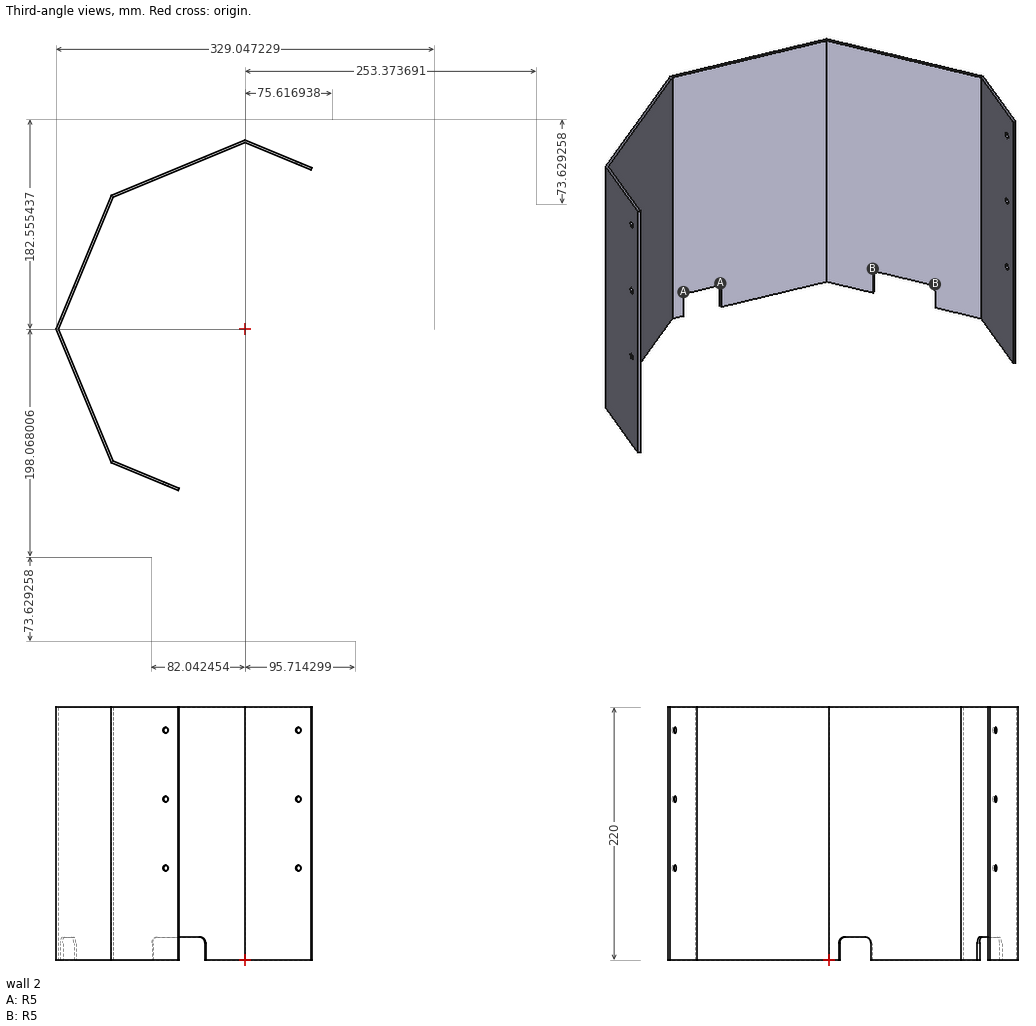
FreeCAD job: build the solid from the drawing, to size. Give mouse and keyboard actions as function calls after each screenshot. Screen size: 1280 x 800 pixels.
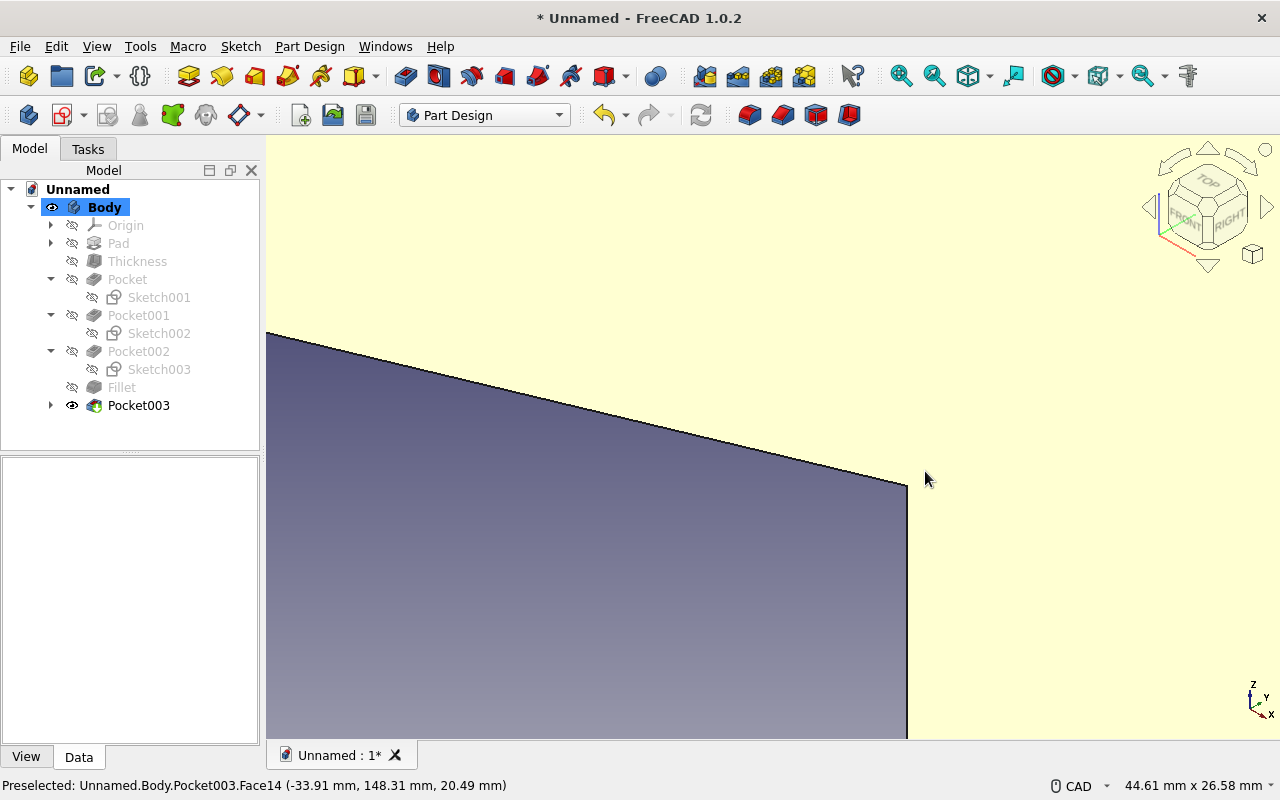
click(902, 76)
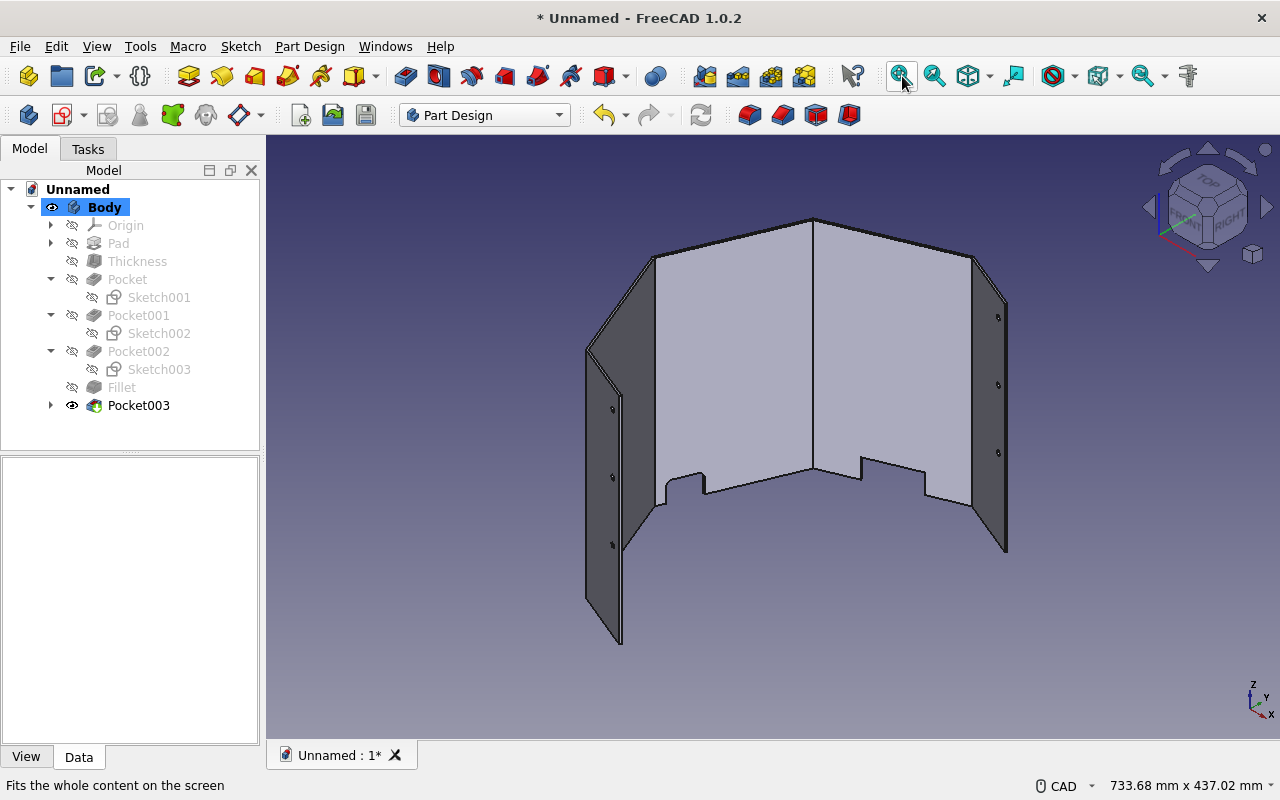
key(2)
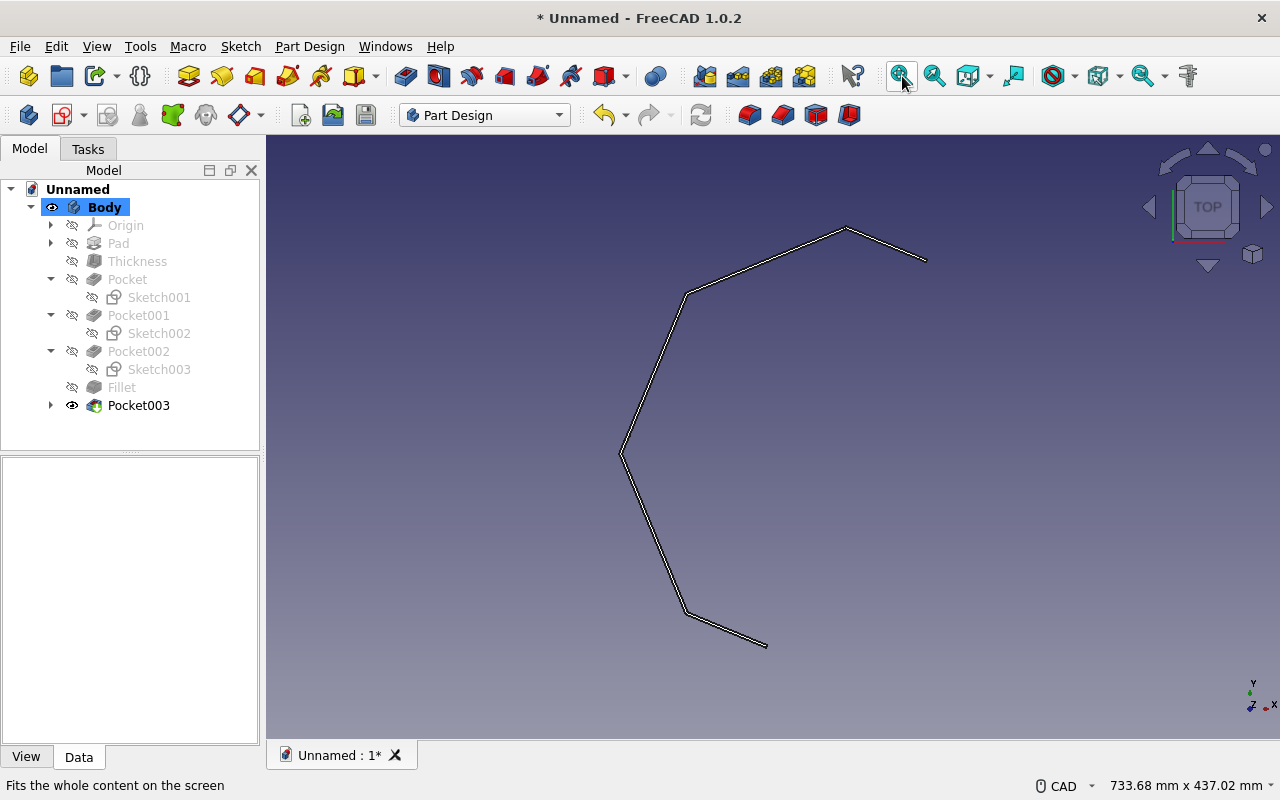
scroll(799, 247, up, 14)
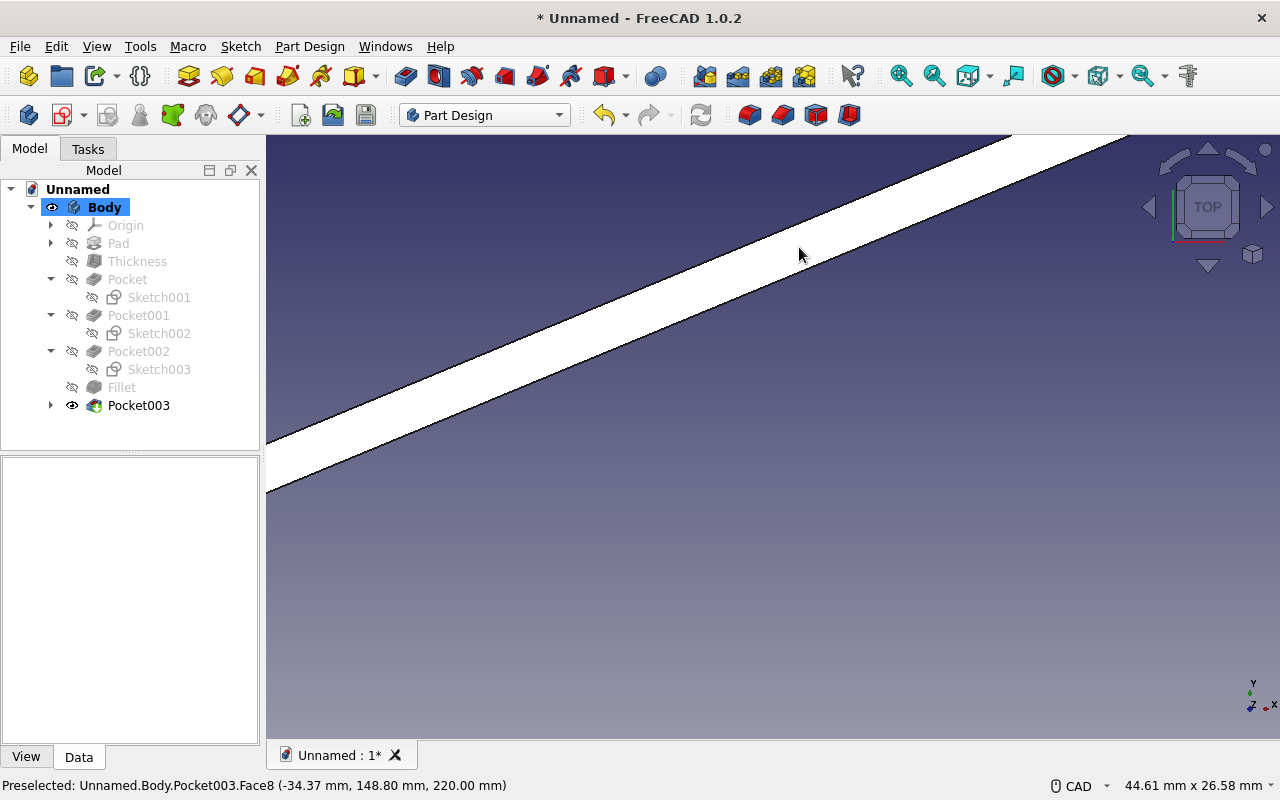
click(902, 76)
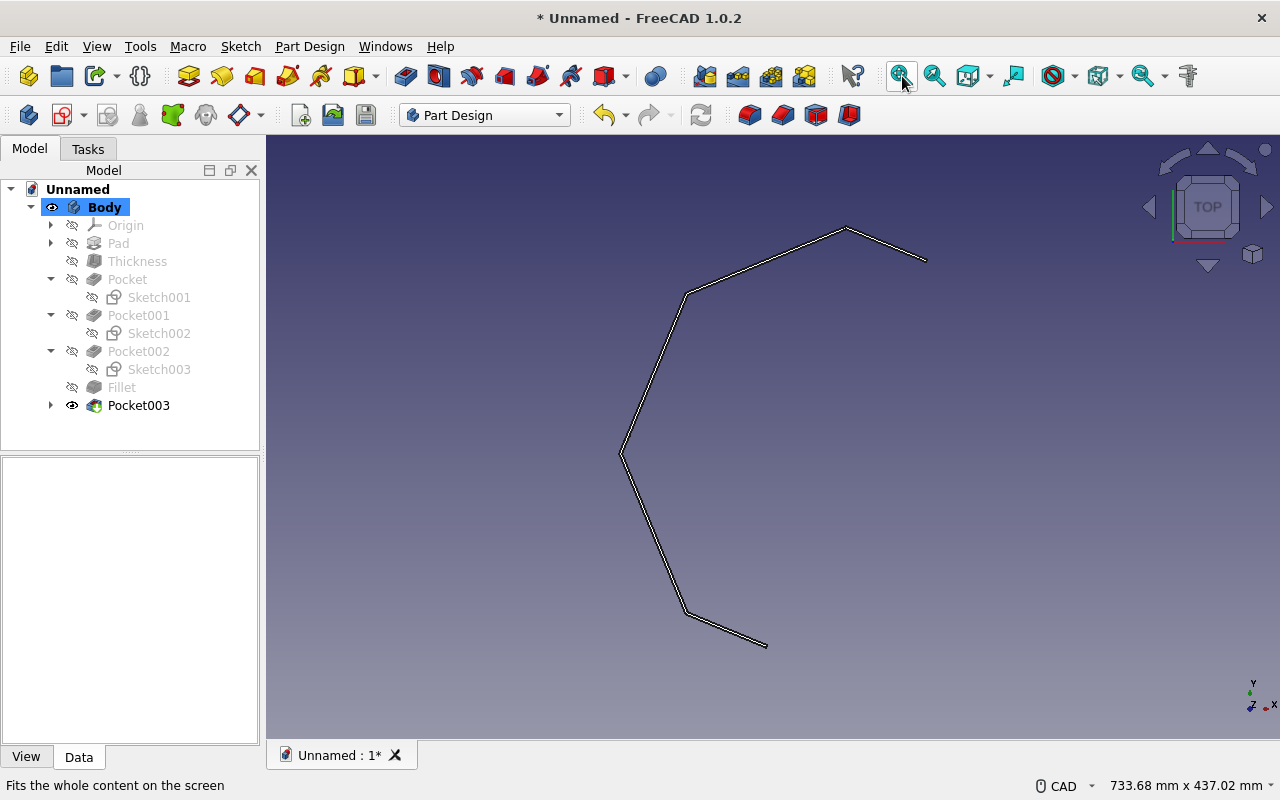
key(1)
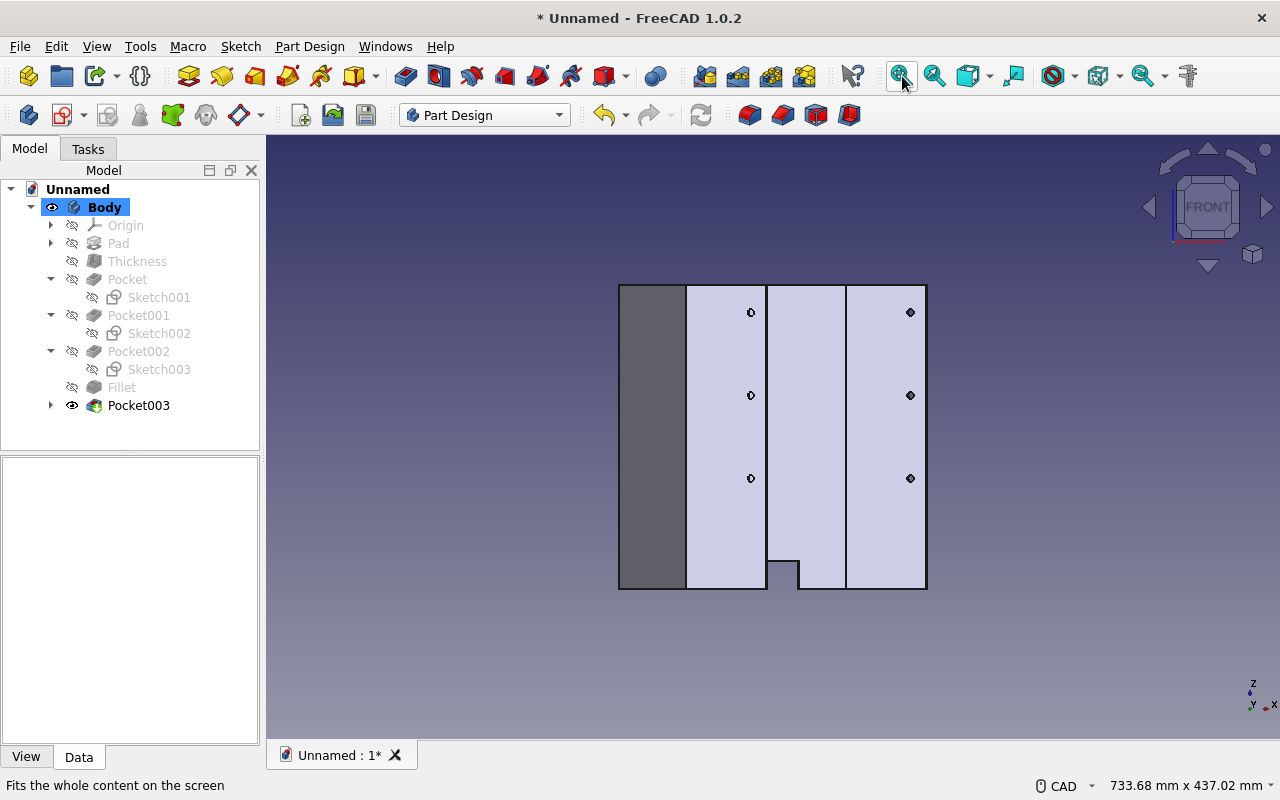
scroll(799, 560, up, 14)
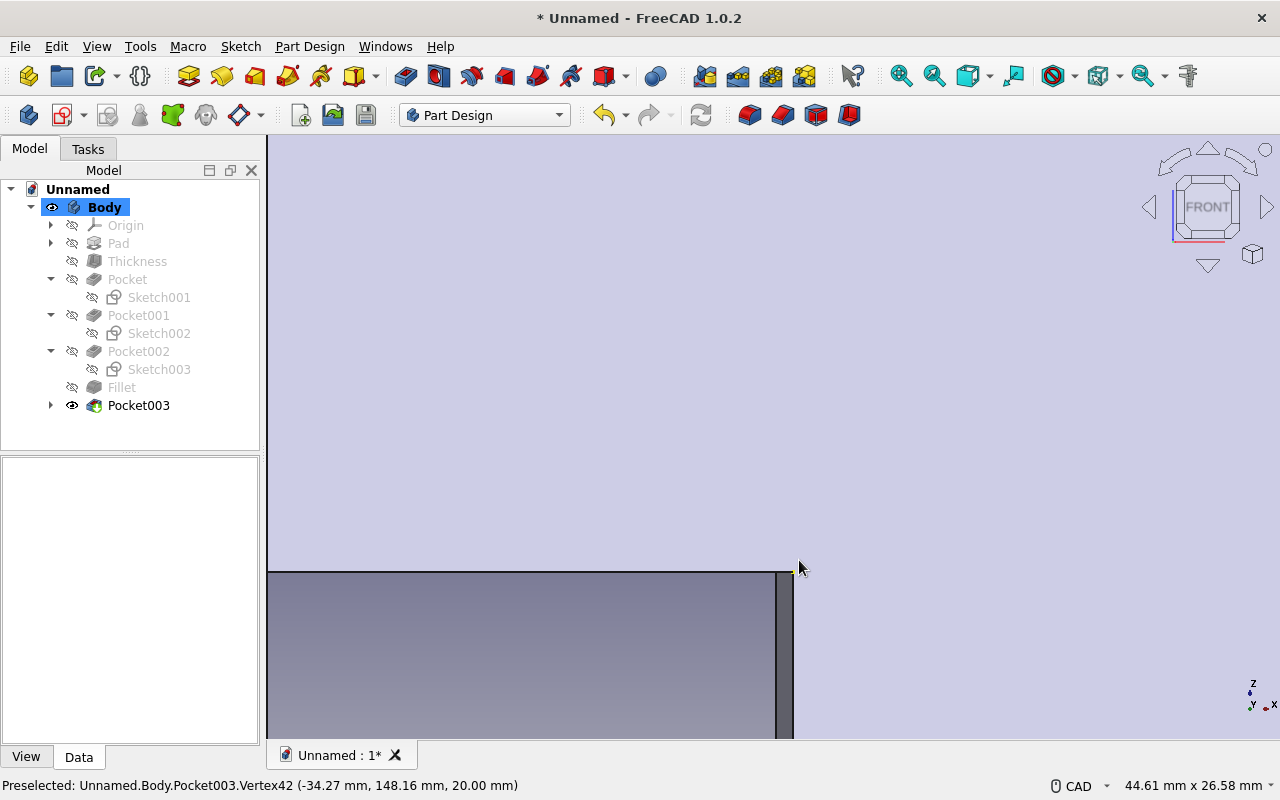
click(902, 76)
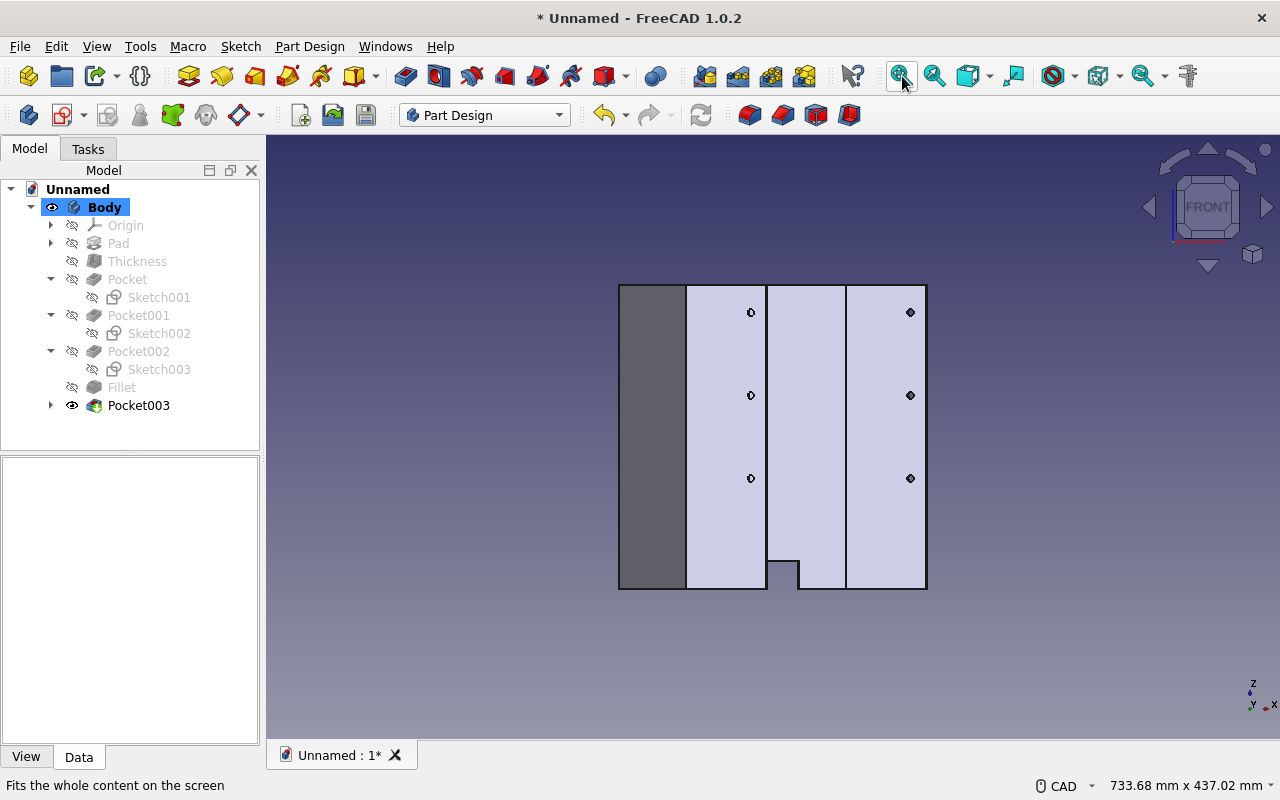
key(3)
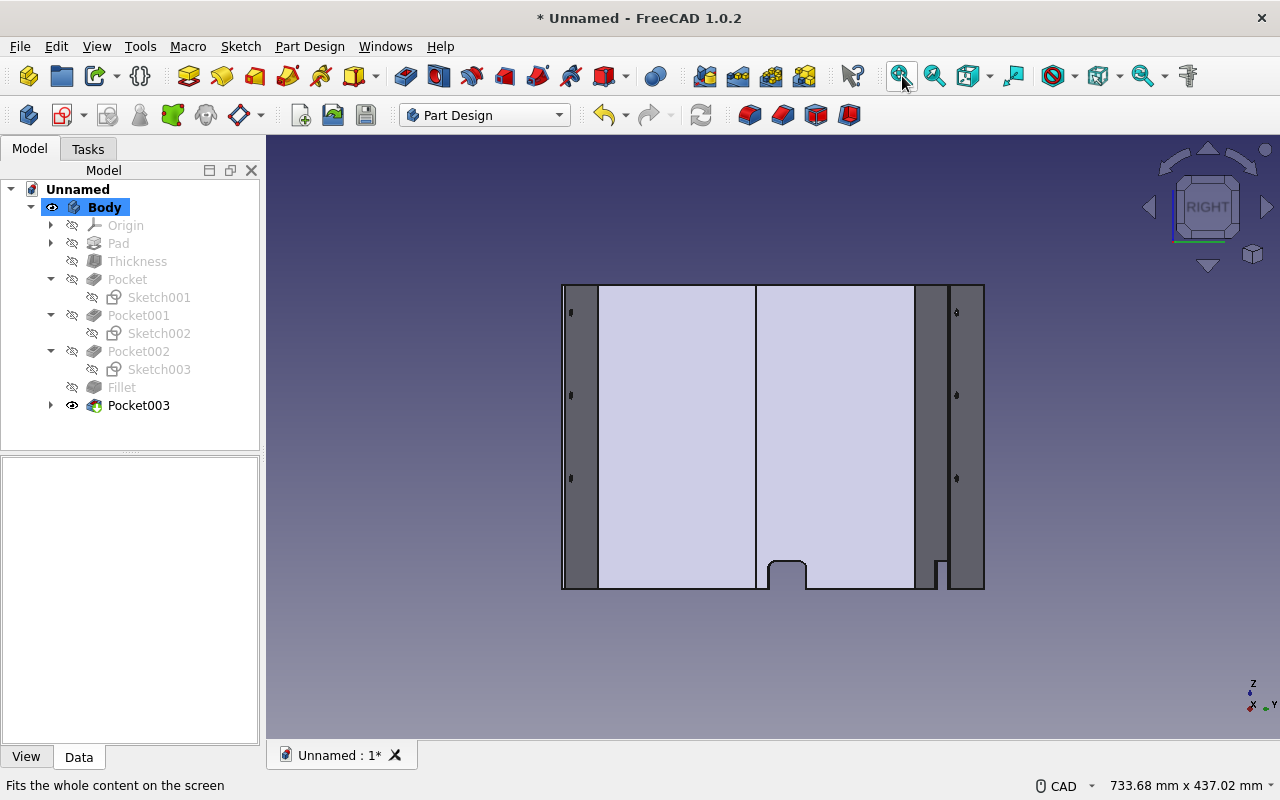
scroll(962, 560, up, 14)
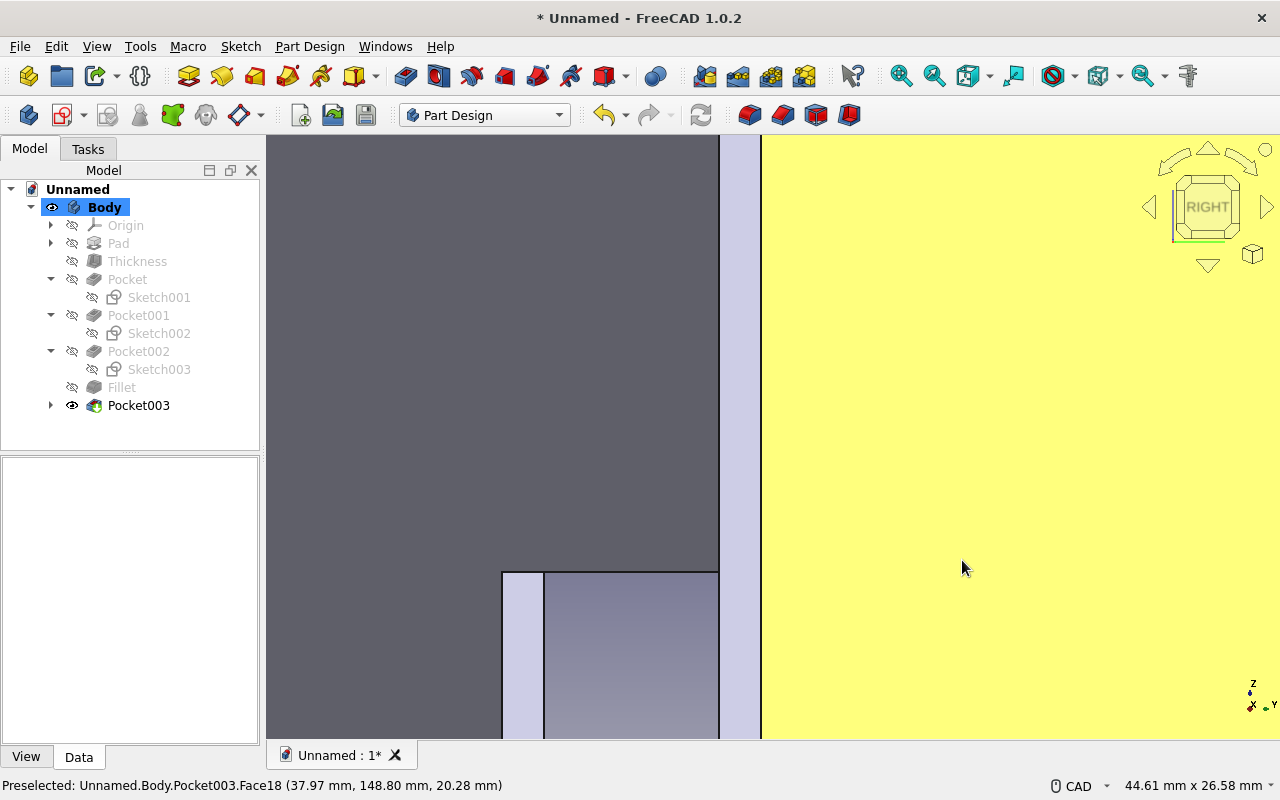
click(902, 76)